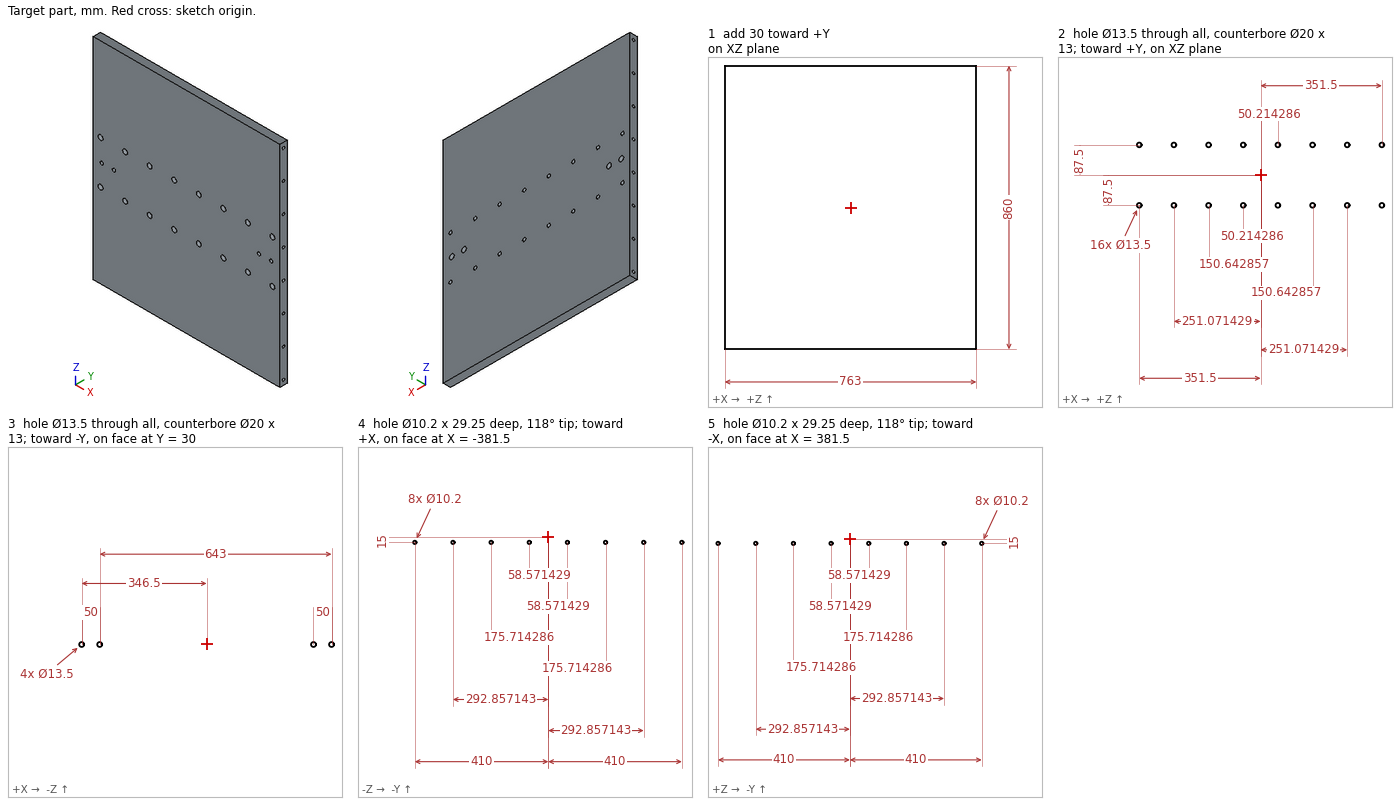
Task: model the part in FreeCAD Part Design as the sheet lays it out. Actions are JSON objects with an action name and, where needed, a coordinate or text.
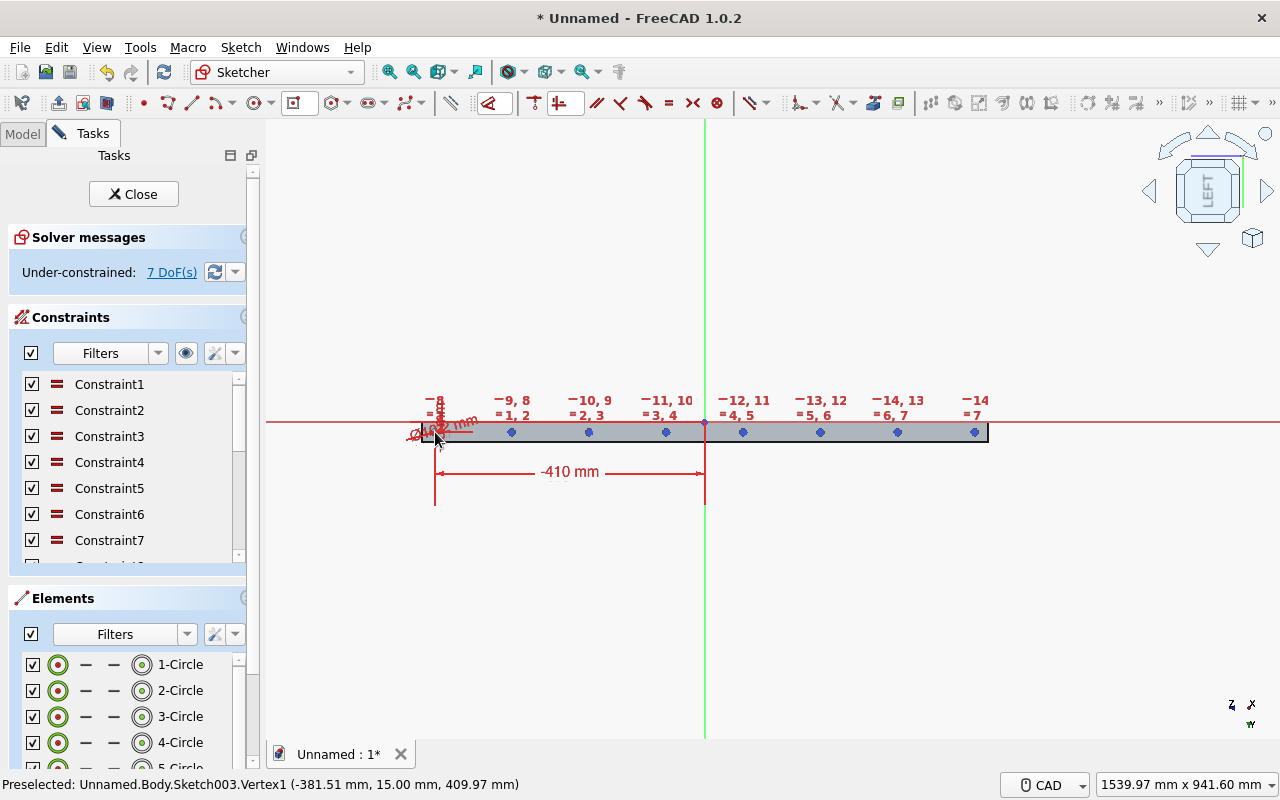
{"action": "left_click", "coordinate": [975, 432]}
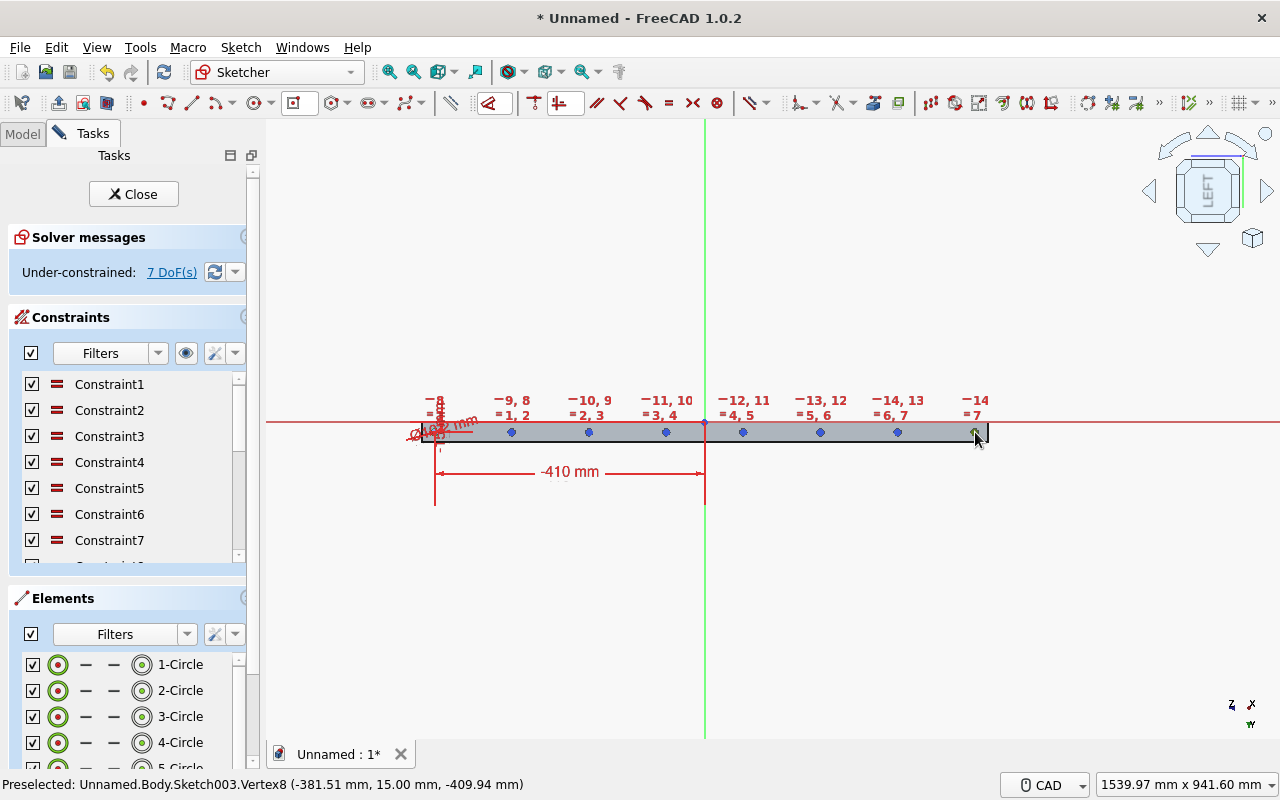
{"action": "left_click", "coordinate": [506, 104]}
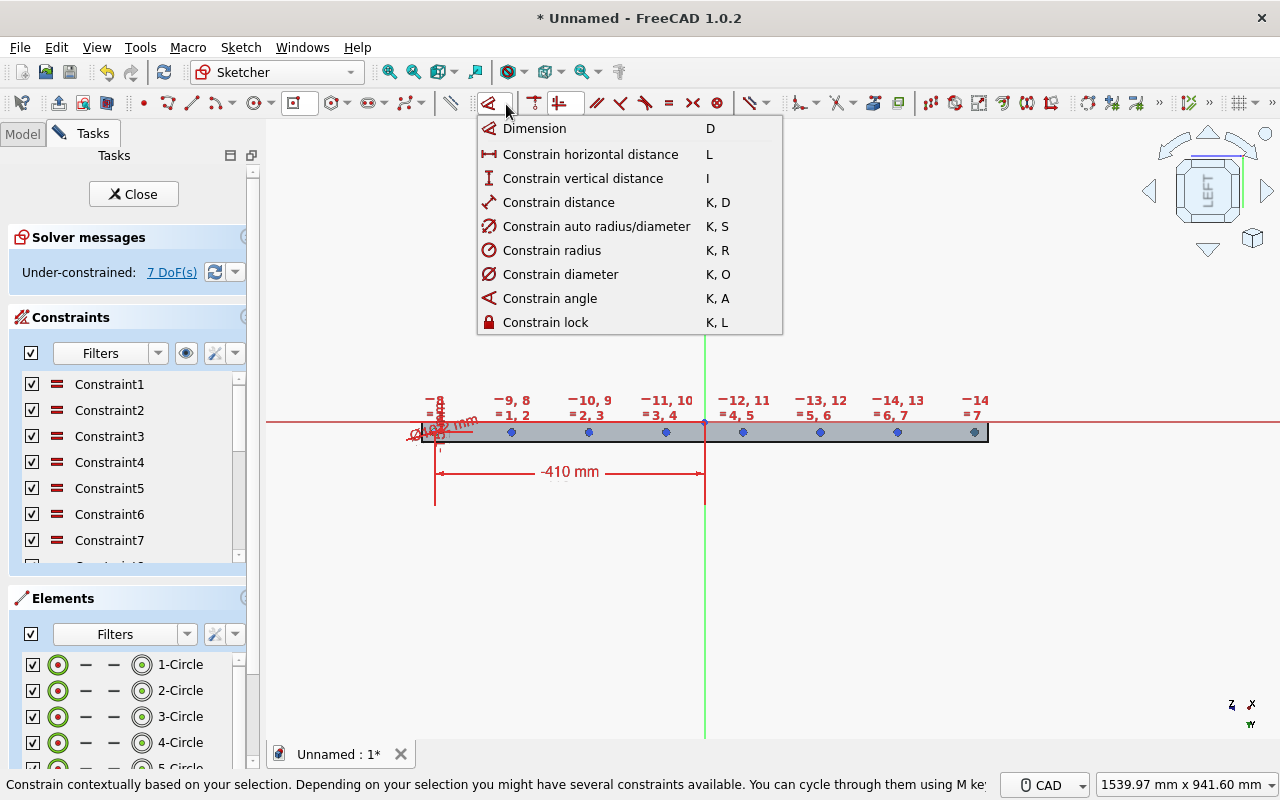
{"action": "left_click", "coordinate": [630, 154]}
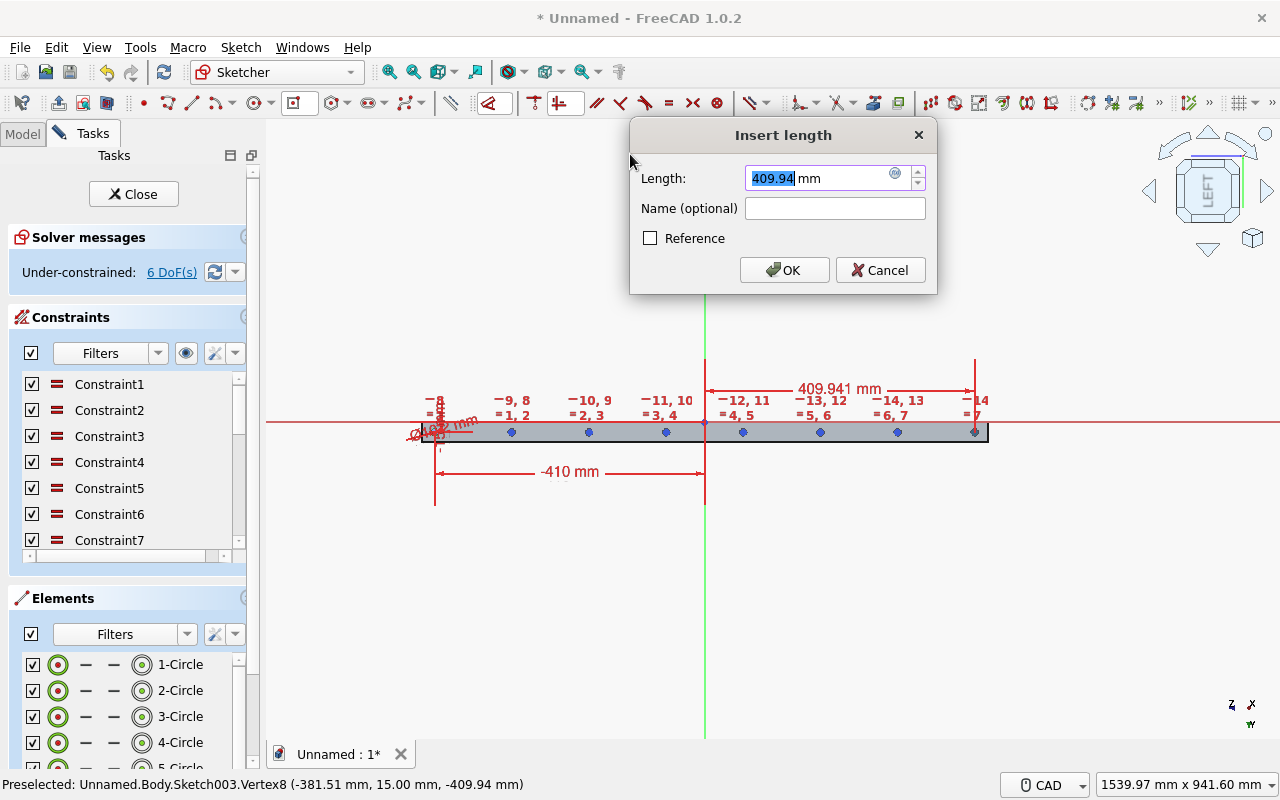
{"action": "type", "text": "410"}
{"action": "key", "text": "Return"}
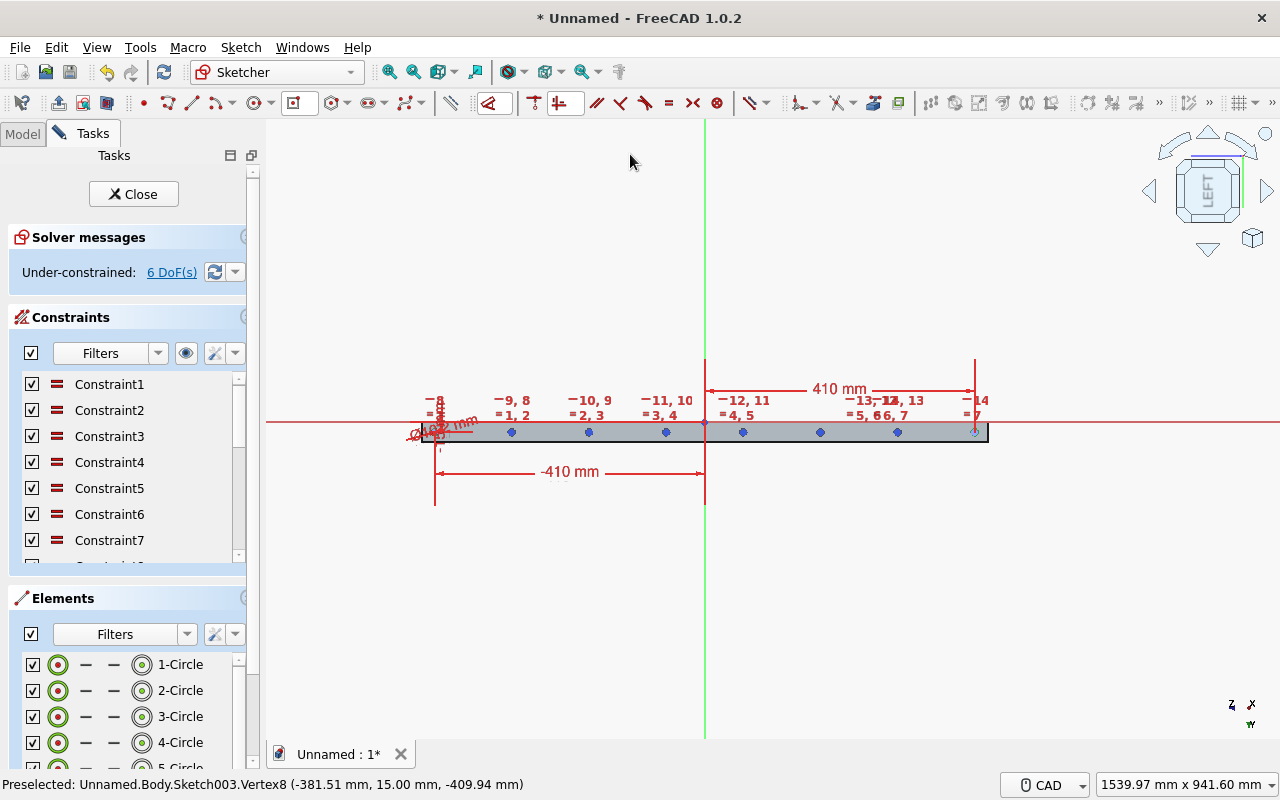
{"action": "left_click", "coordinate": [666, 432]}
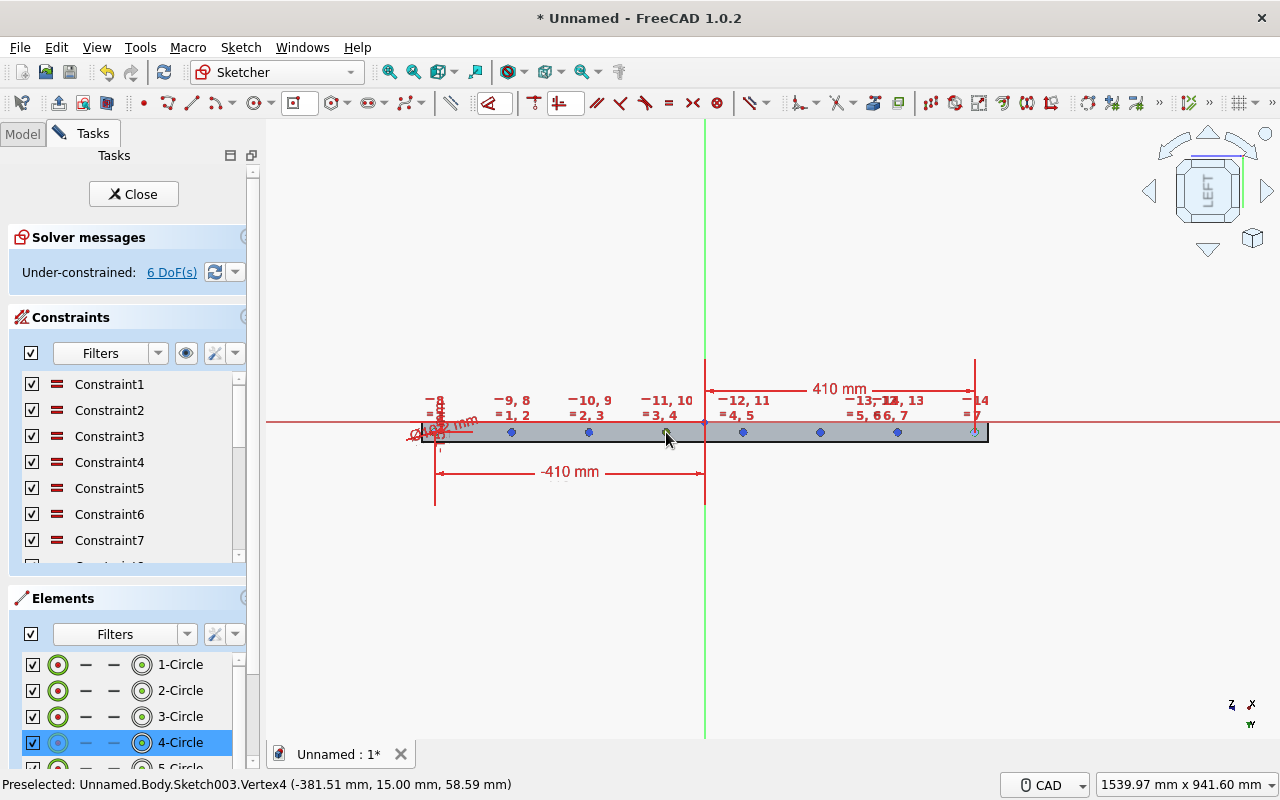
{"action": "left_click", "coordinate": [506, 104]}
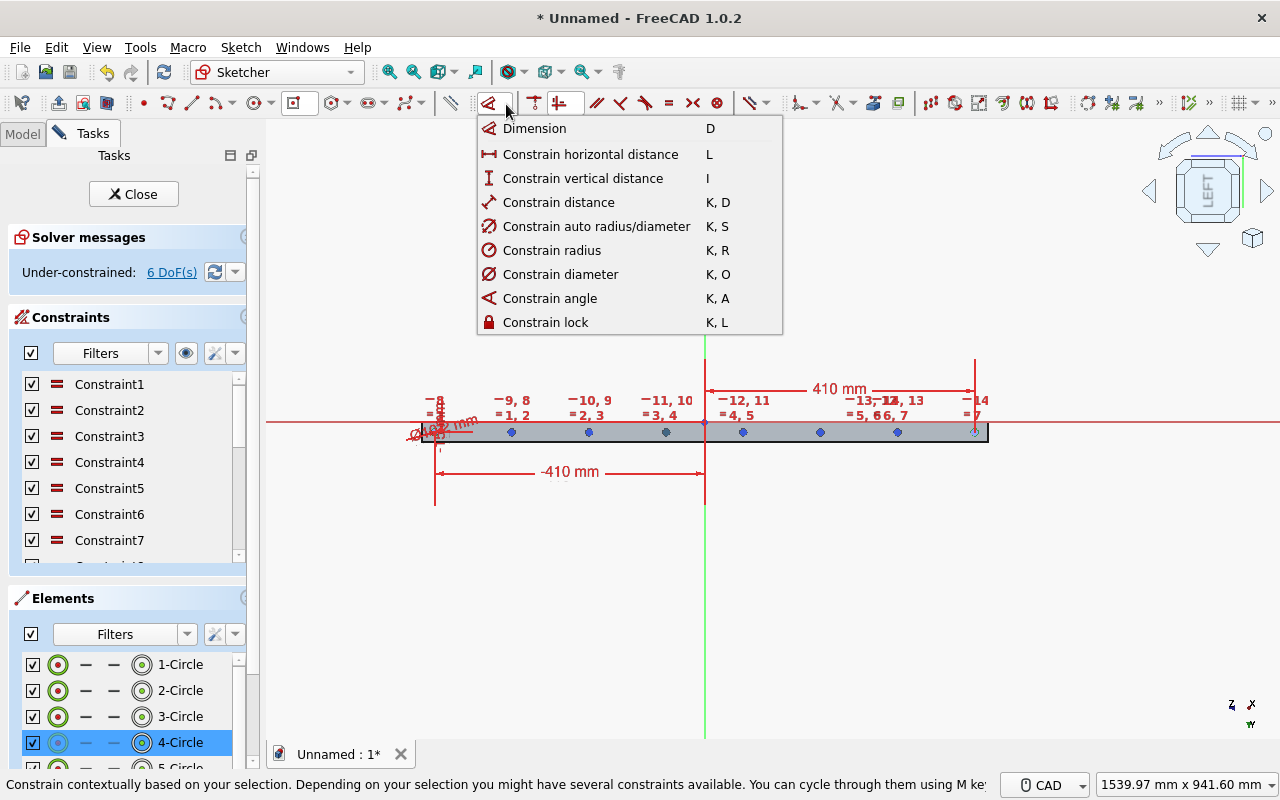
{"action": "left_click", "coordinate": [630, 154]}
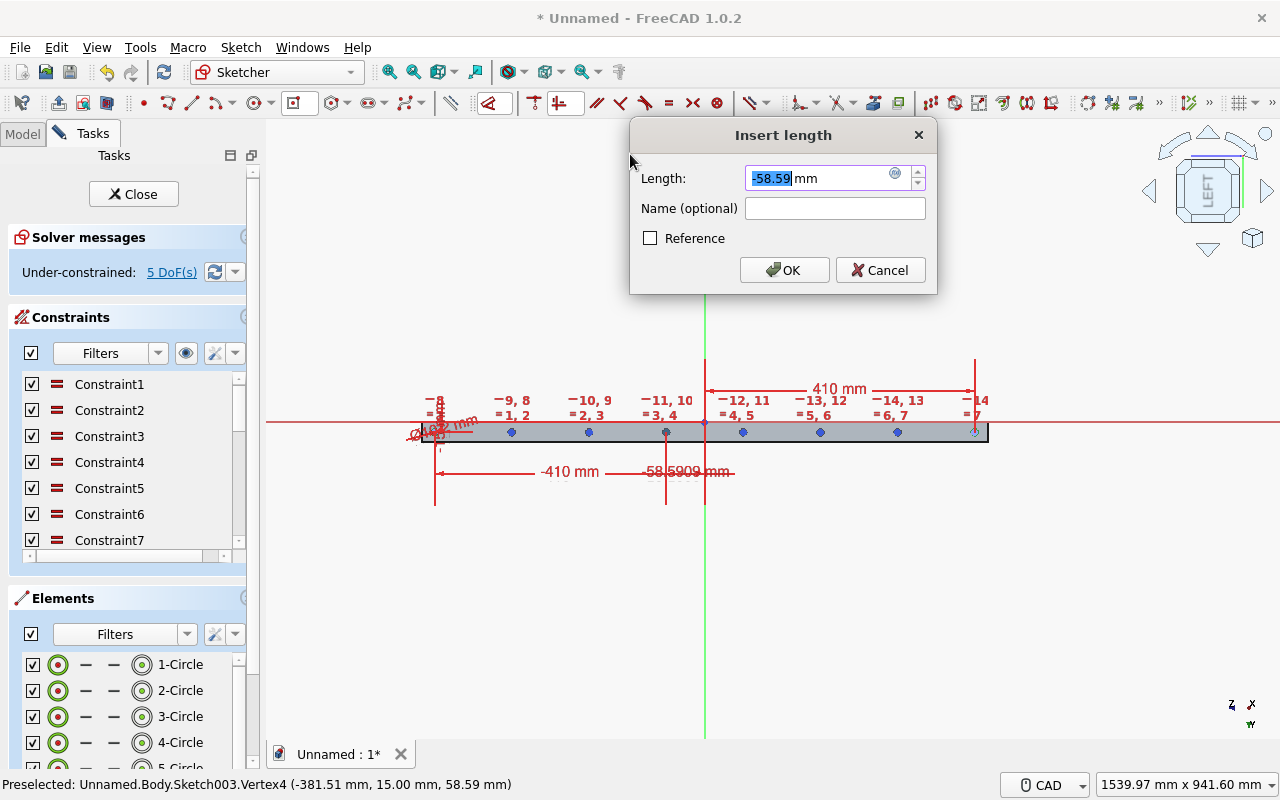
{"action": "type", "text": "-58.571429"}
{"action": "key", "text": "Return"}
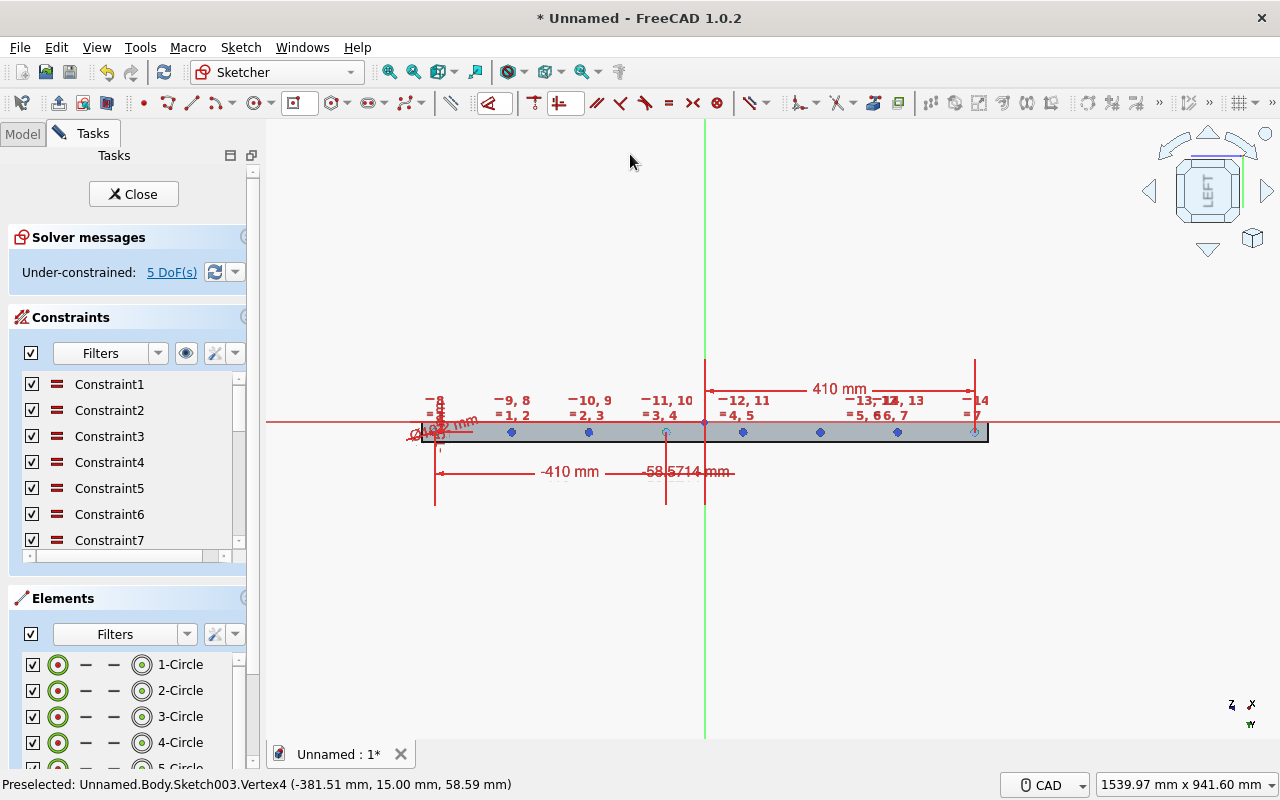
{"action": "left_click", "coordinate": [743, 432]}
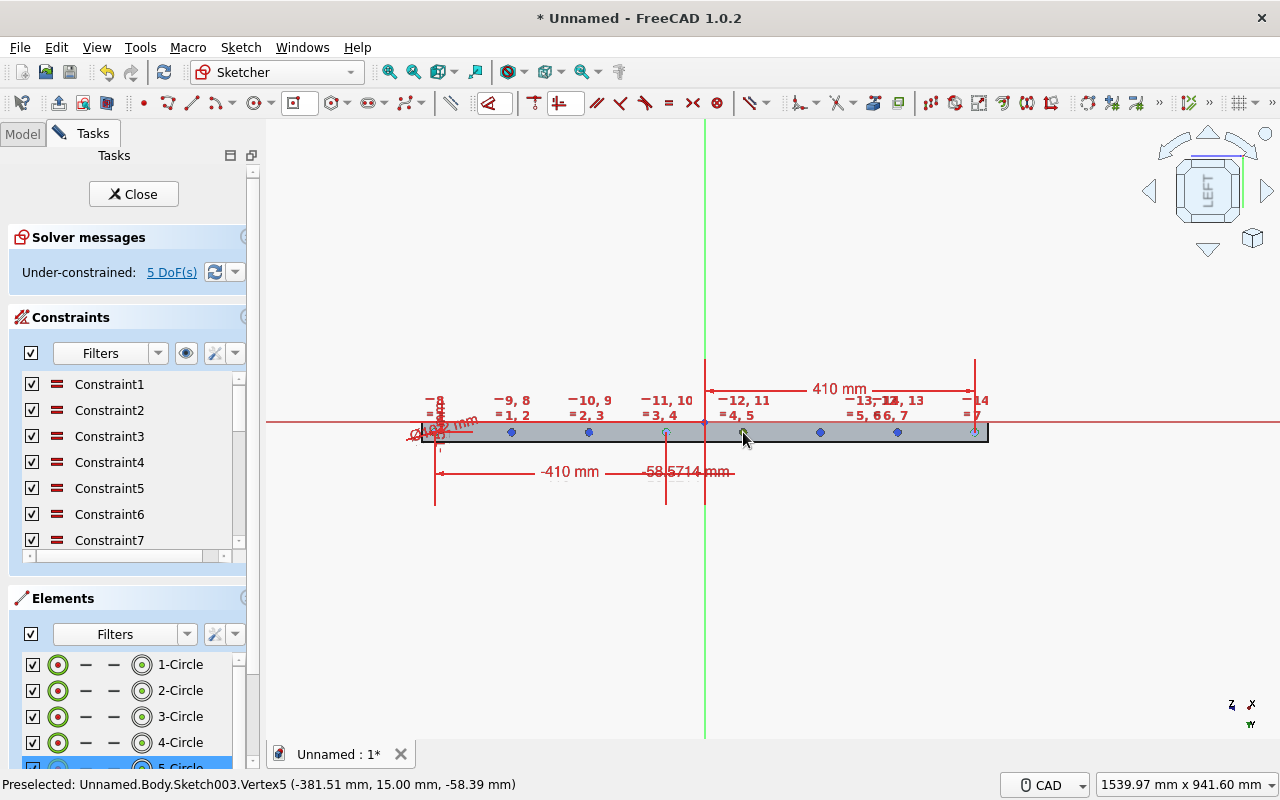
{"action": "left_click", "coordinate": [506, 104]}